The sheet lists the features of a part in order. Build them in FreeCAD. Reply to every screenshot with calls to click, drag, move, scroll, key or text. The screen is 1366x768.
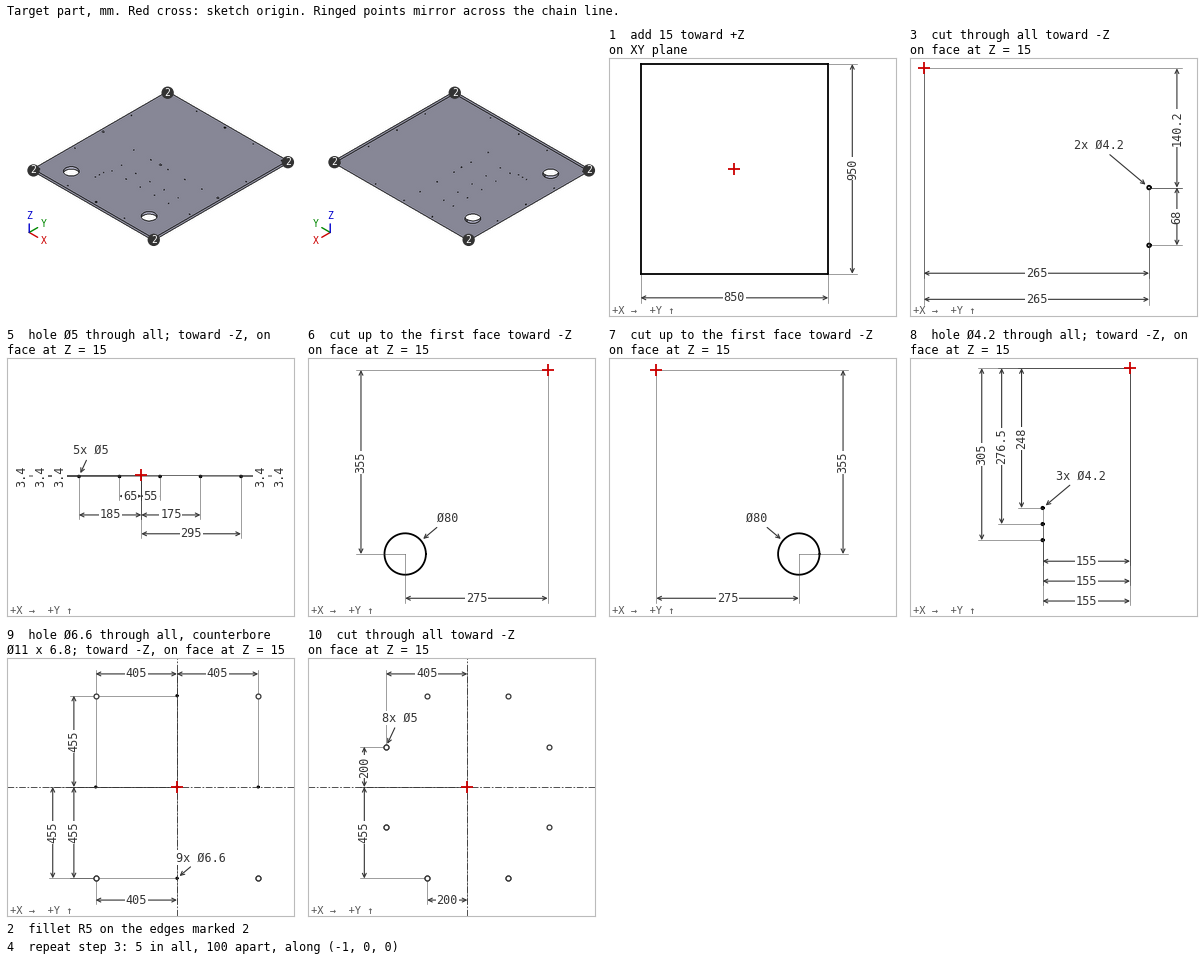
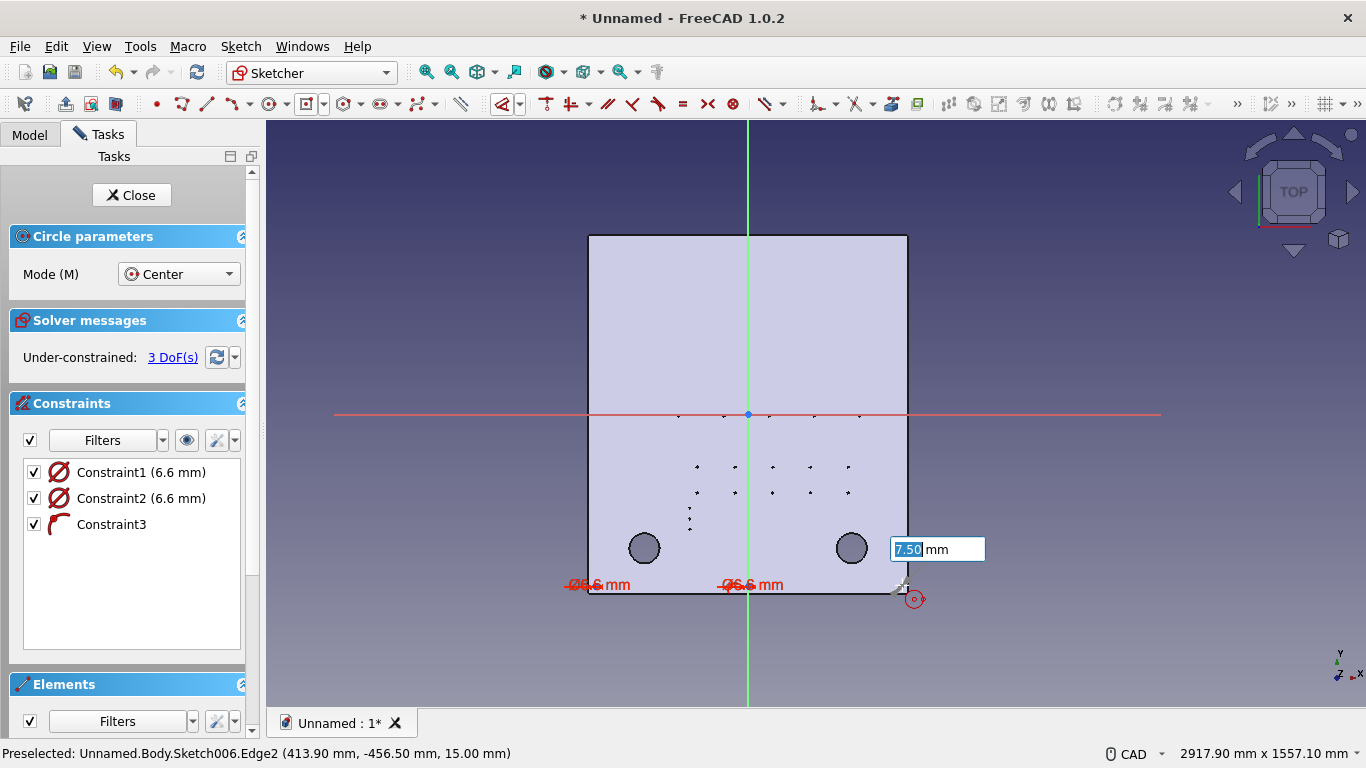
text(6.6)
key(Return)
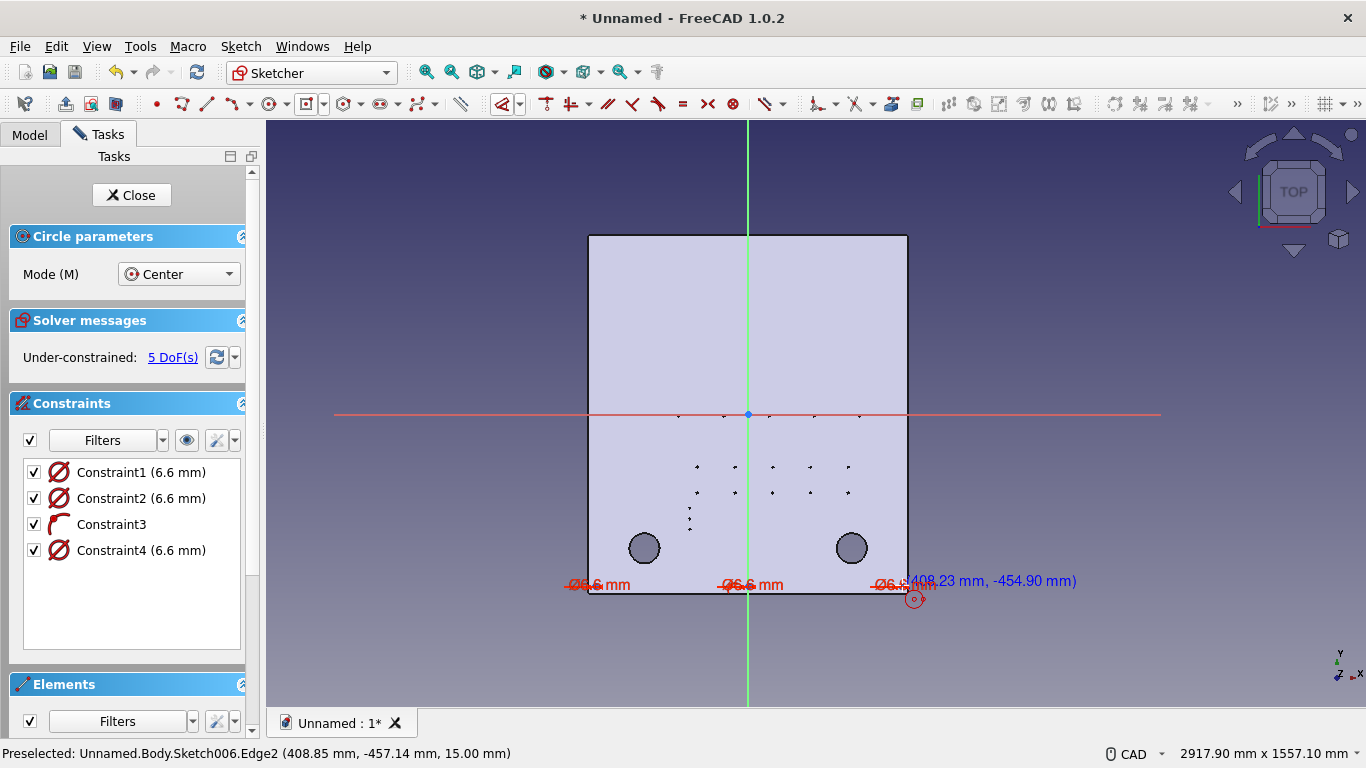
scroll(748, 415, up, 15)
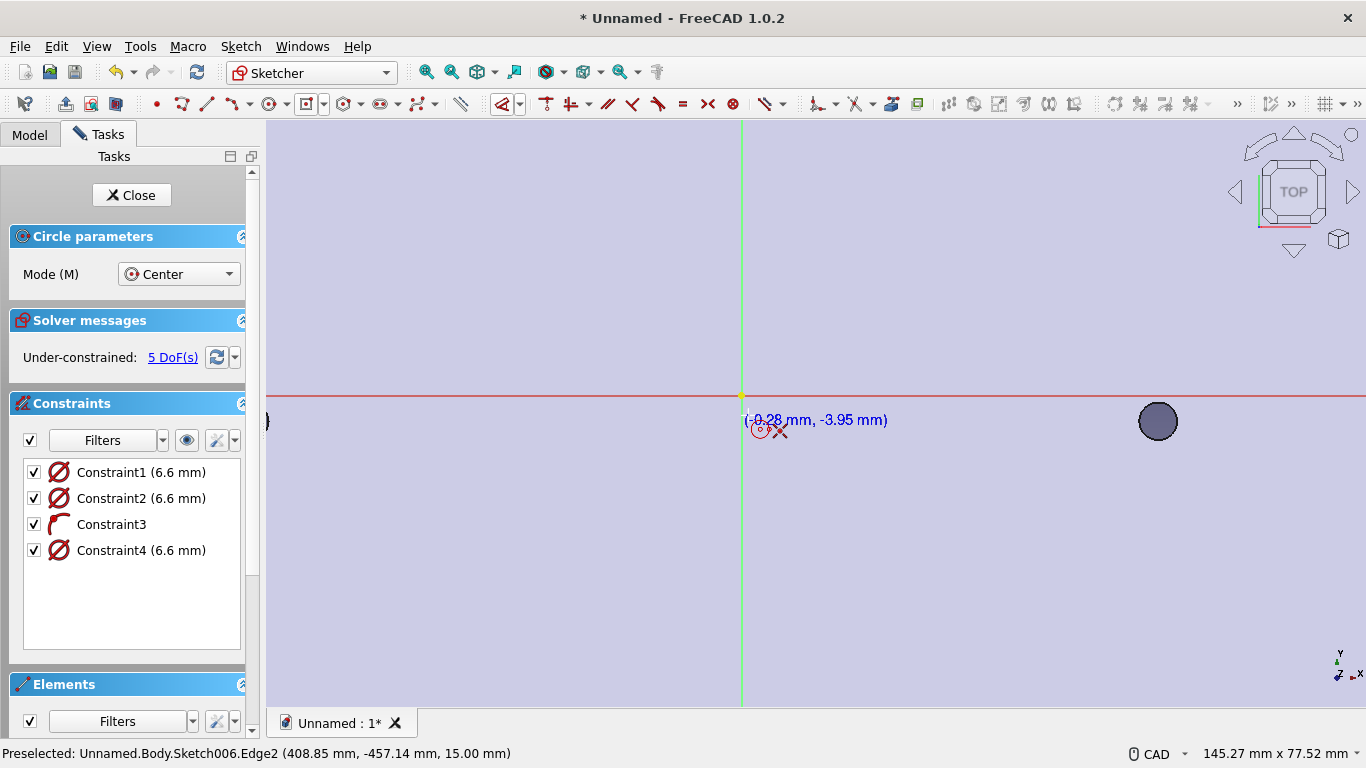
scroll(748, 414, down, 15)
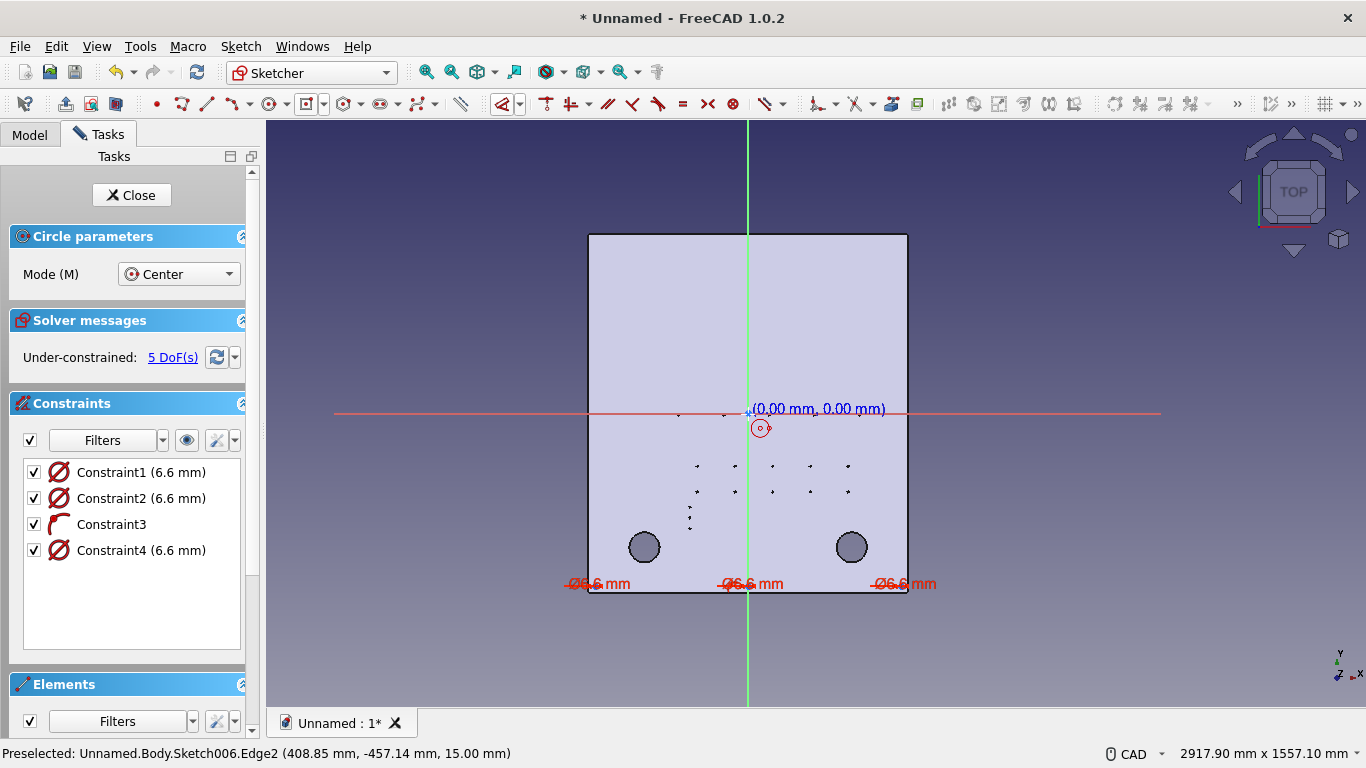
click(748, 414)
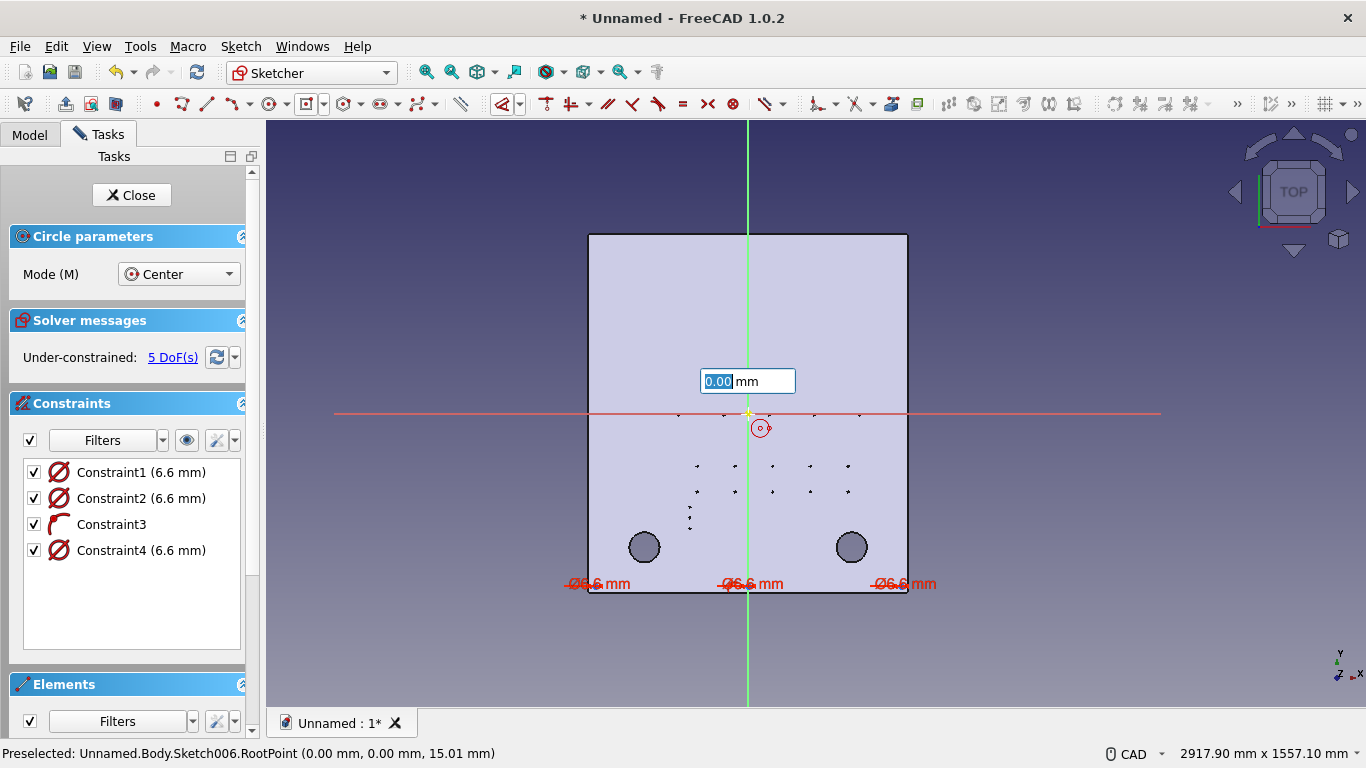
scroll(749, 413, up, 15)
move(740, 397)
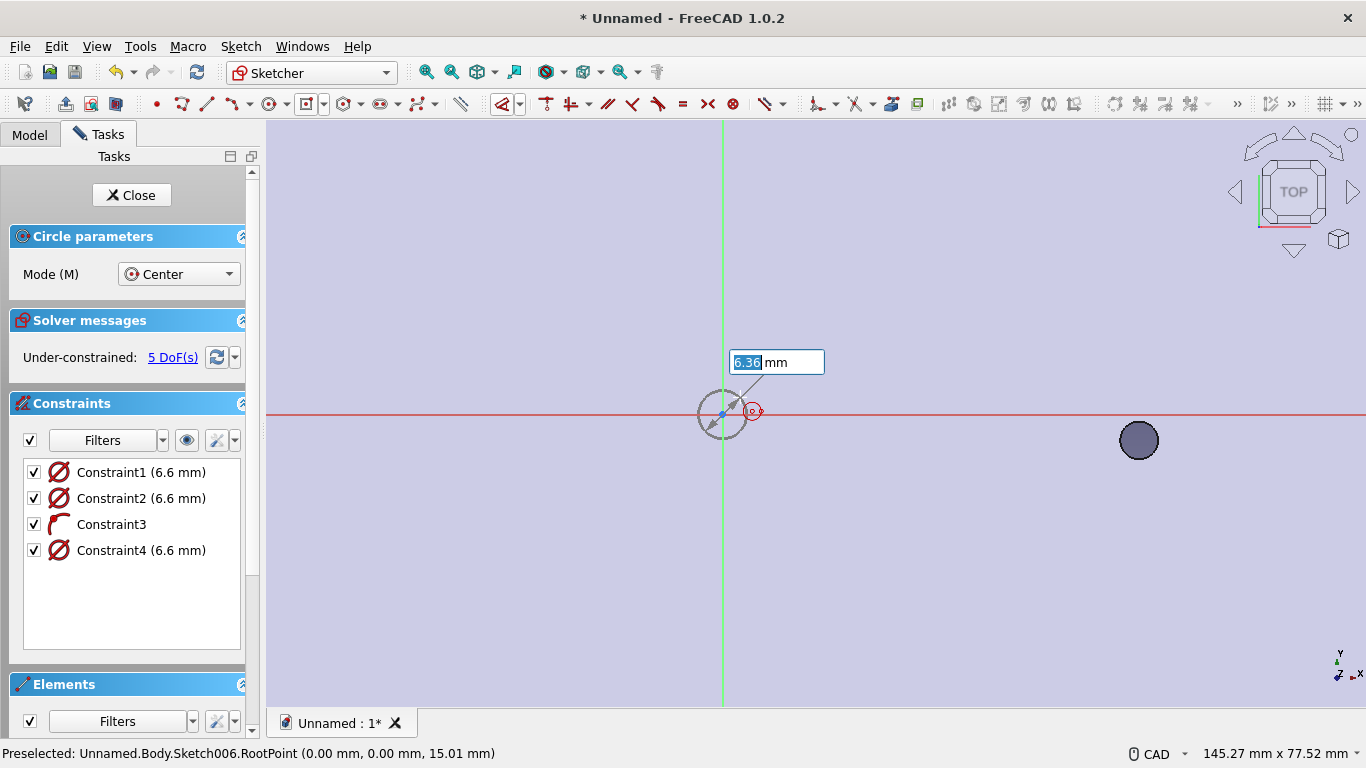
text(6.6)
key(Return)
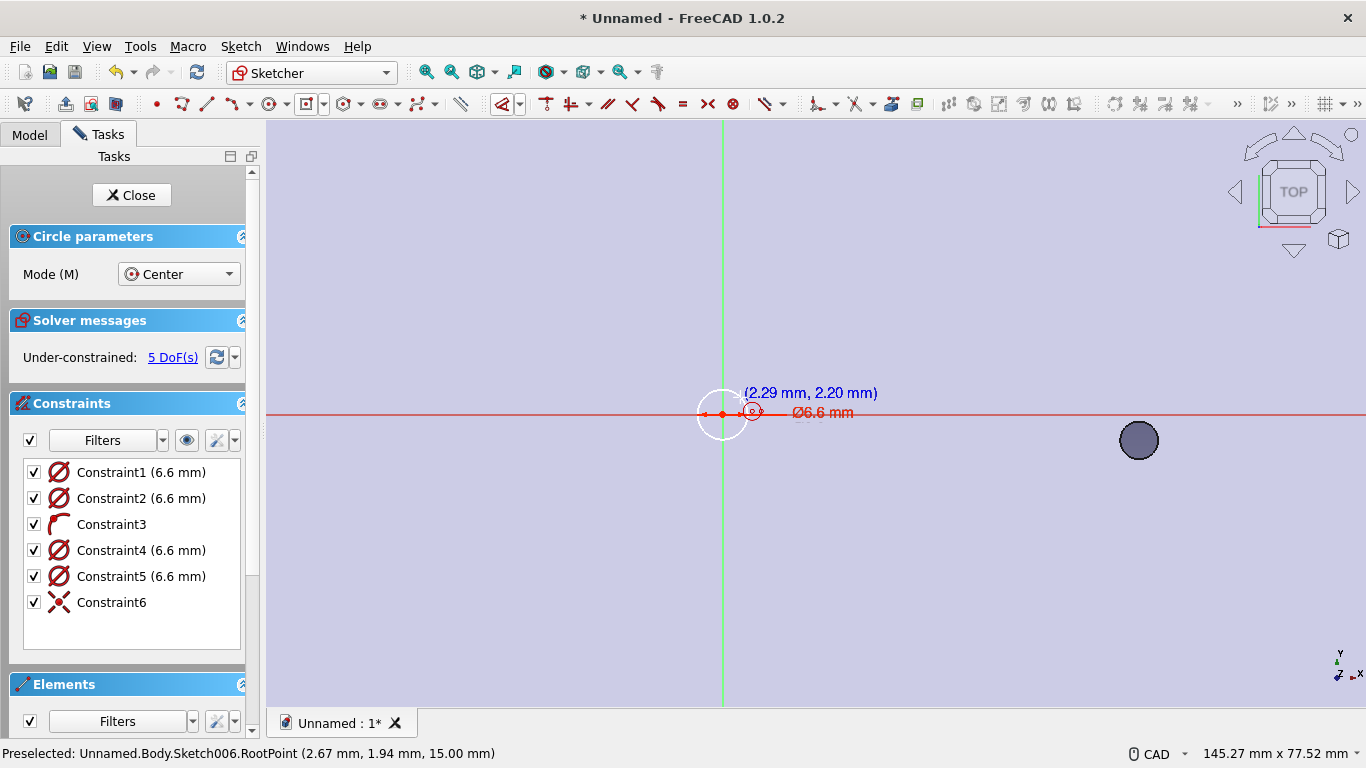
scroll(749, 413, down, 15)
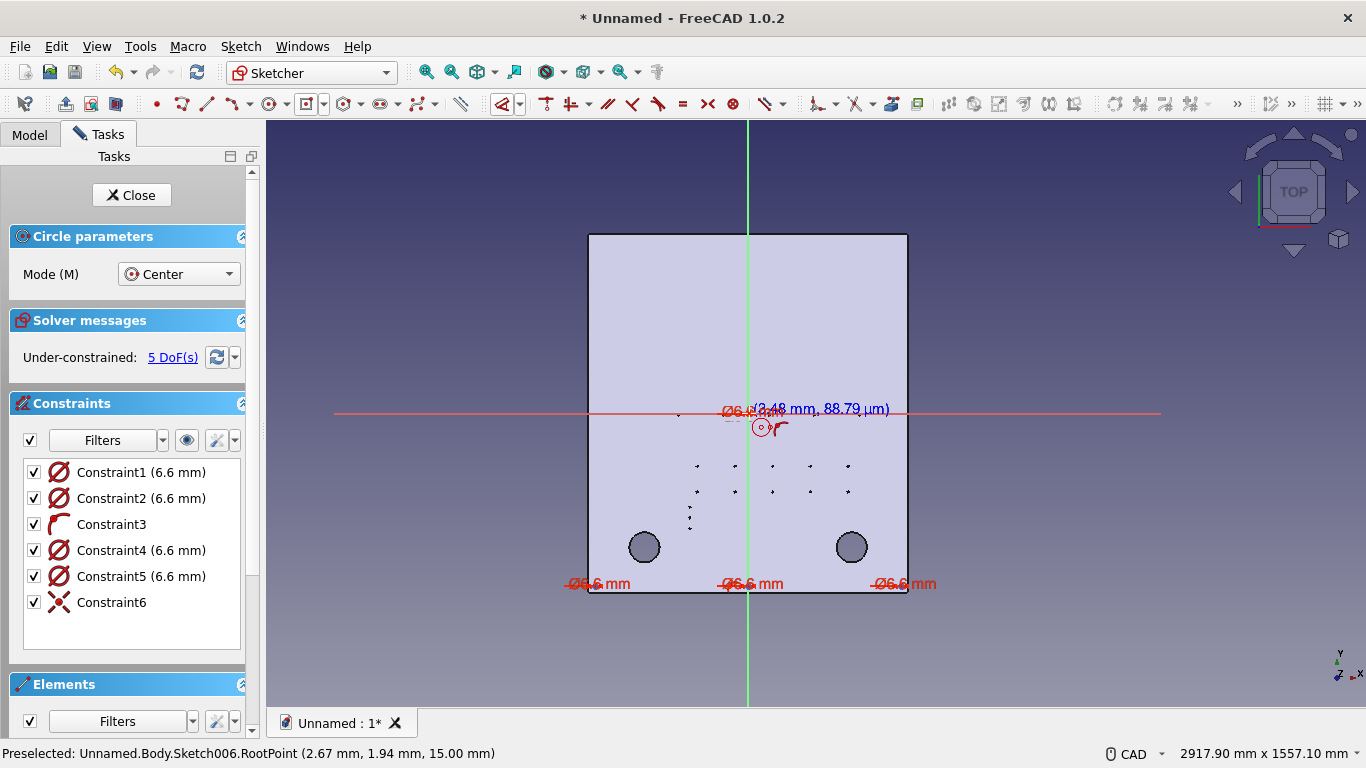
scroll(595, 414, up, 15)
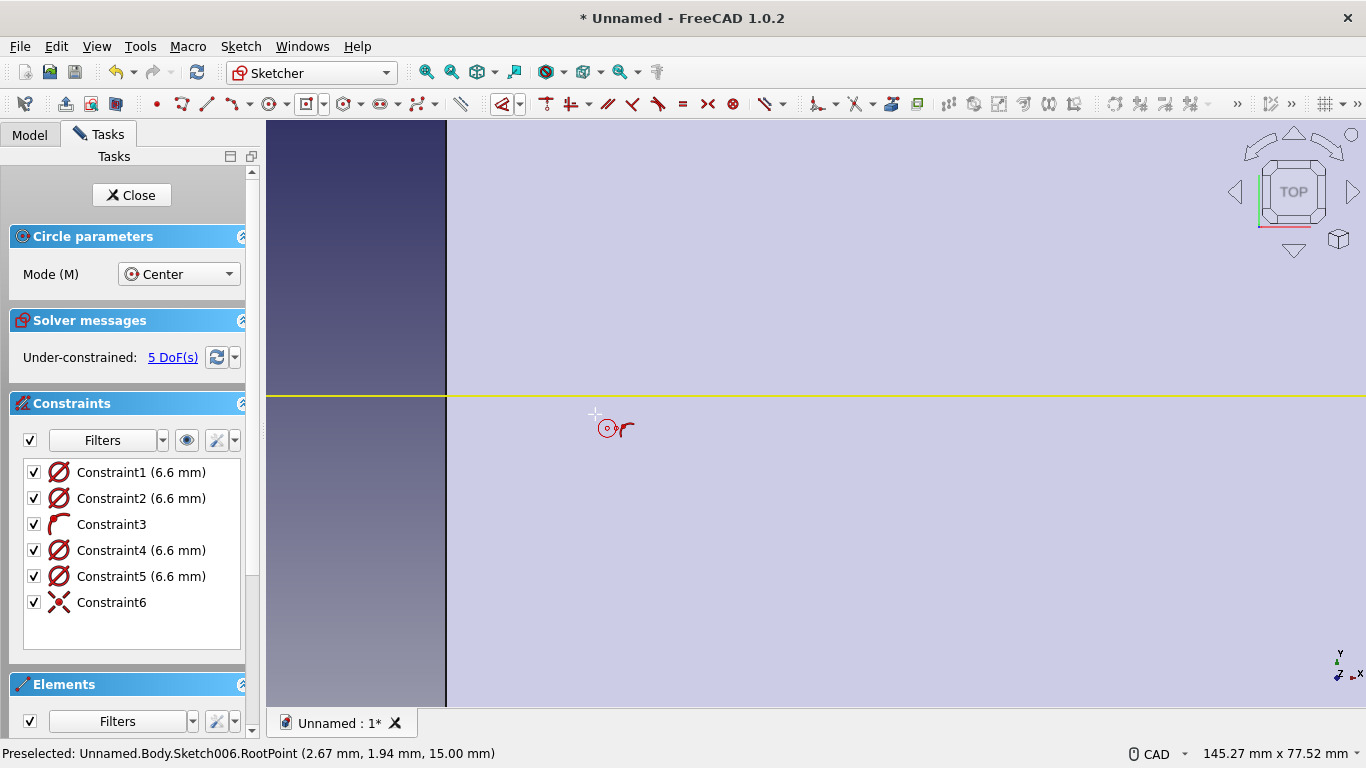
scroll(595, 414, down, 15)